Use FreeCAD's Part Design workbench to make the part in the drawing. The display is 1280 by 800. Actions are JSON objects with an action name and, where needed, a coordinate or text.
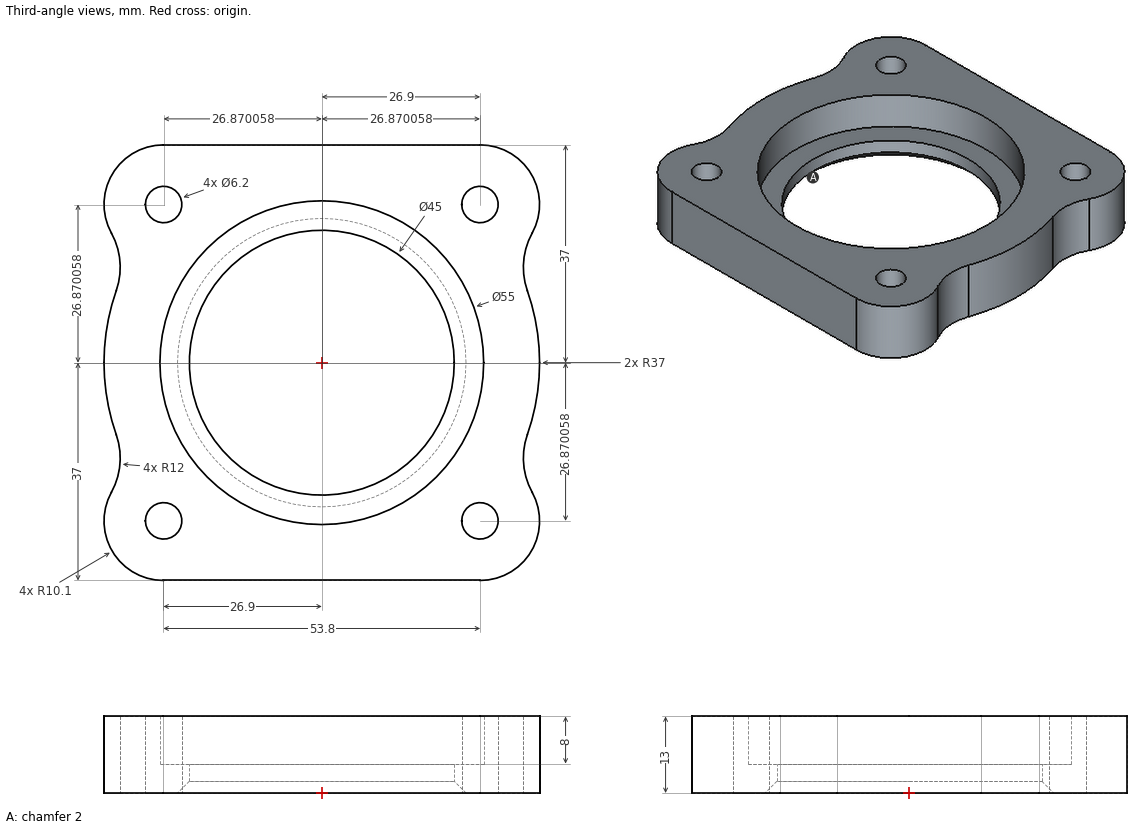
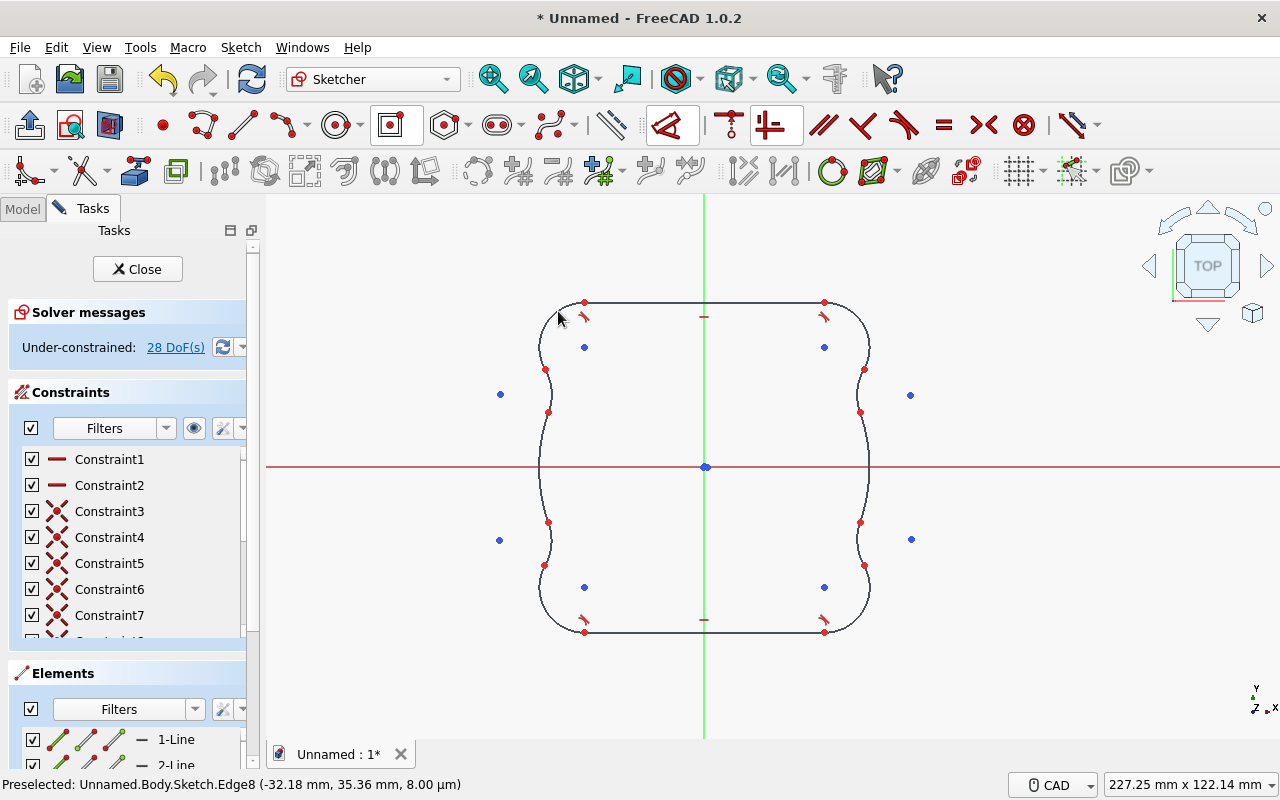
{"action": "left_click", "coordinate": [851, 624]}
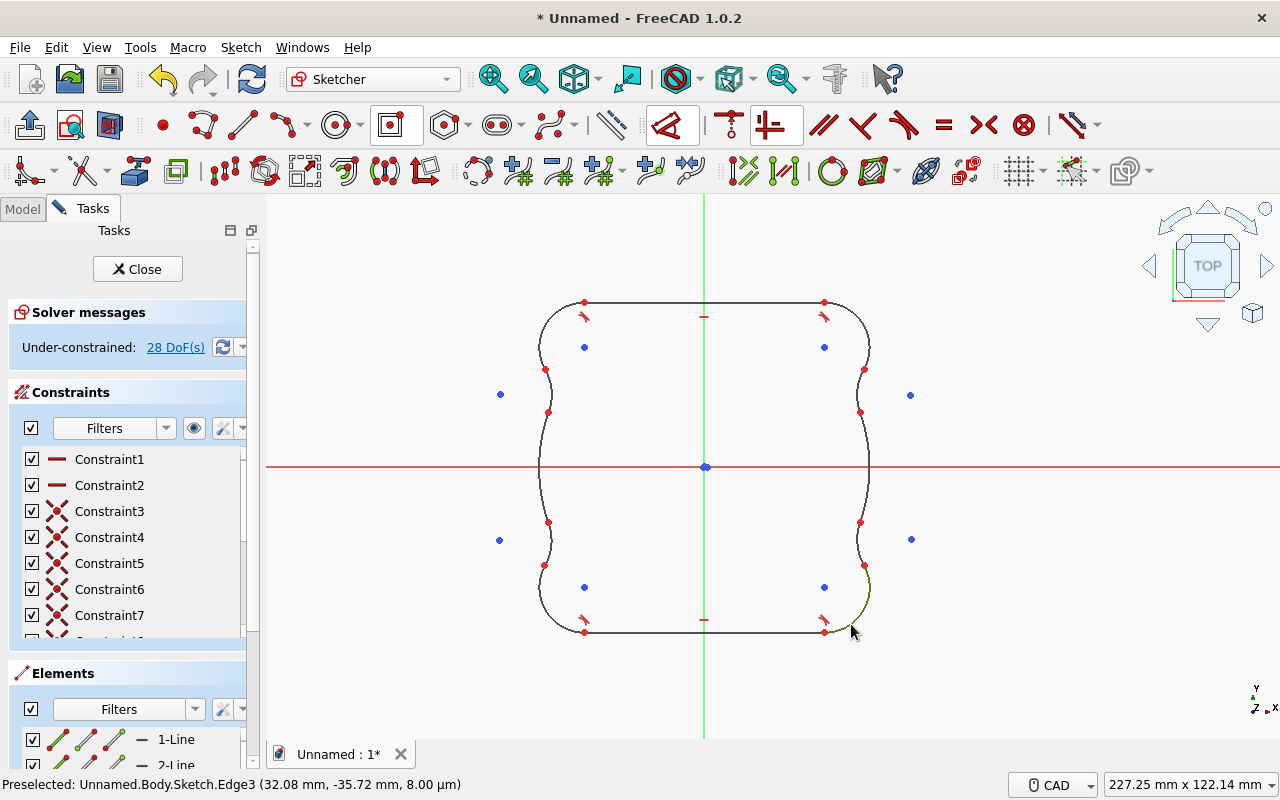
{"action": "left_click", "coordinate": [857, 535]}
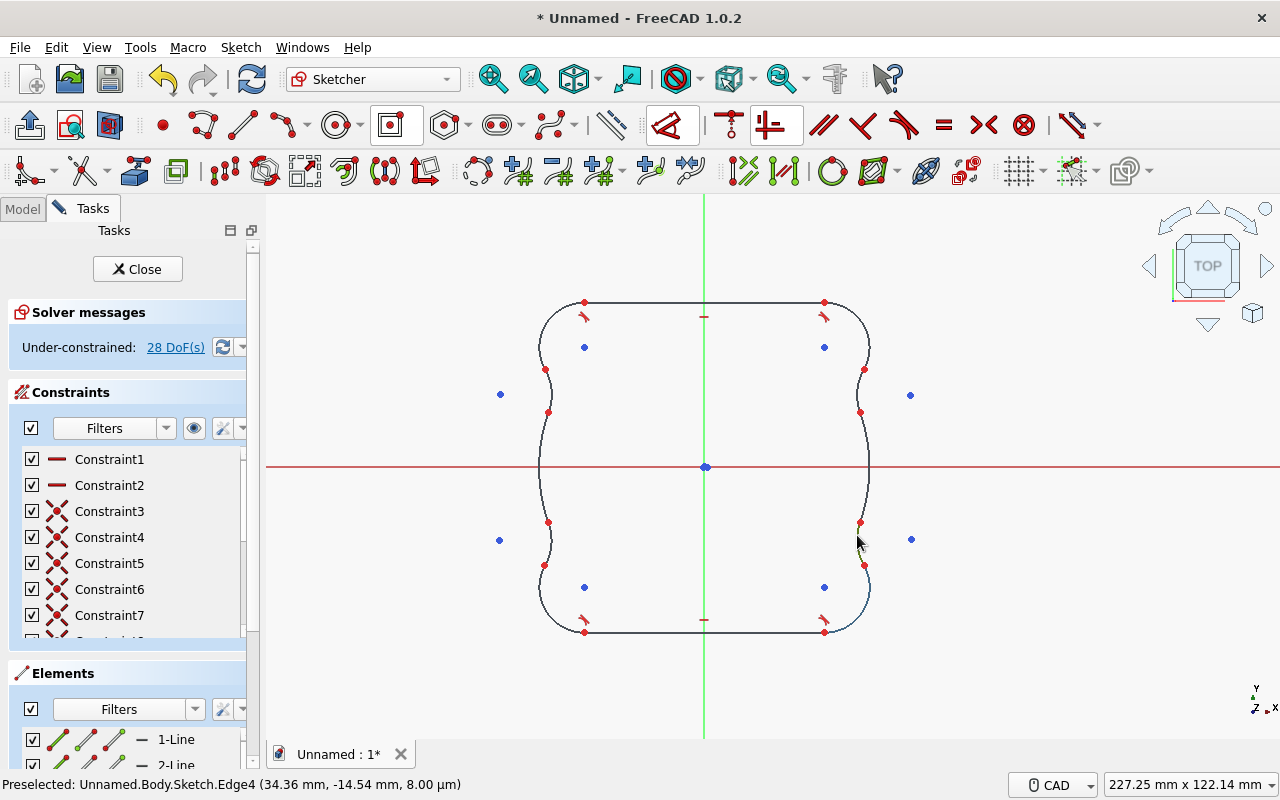
{"action": "key", "text": "t"}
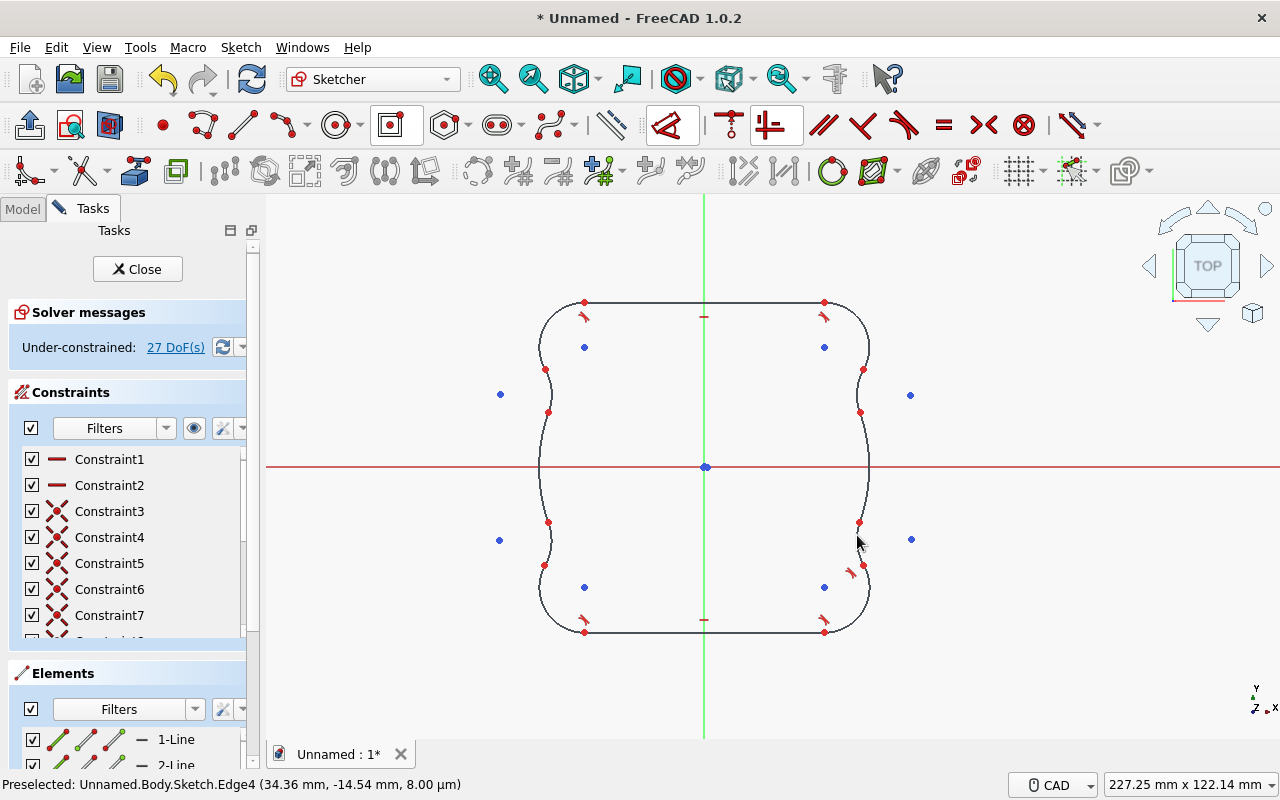
{"action": "left_click", "coordinate": [857, 535]}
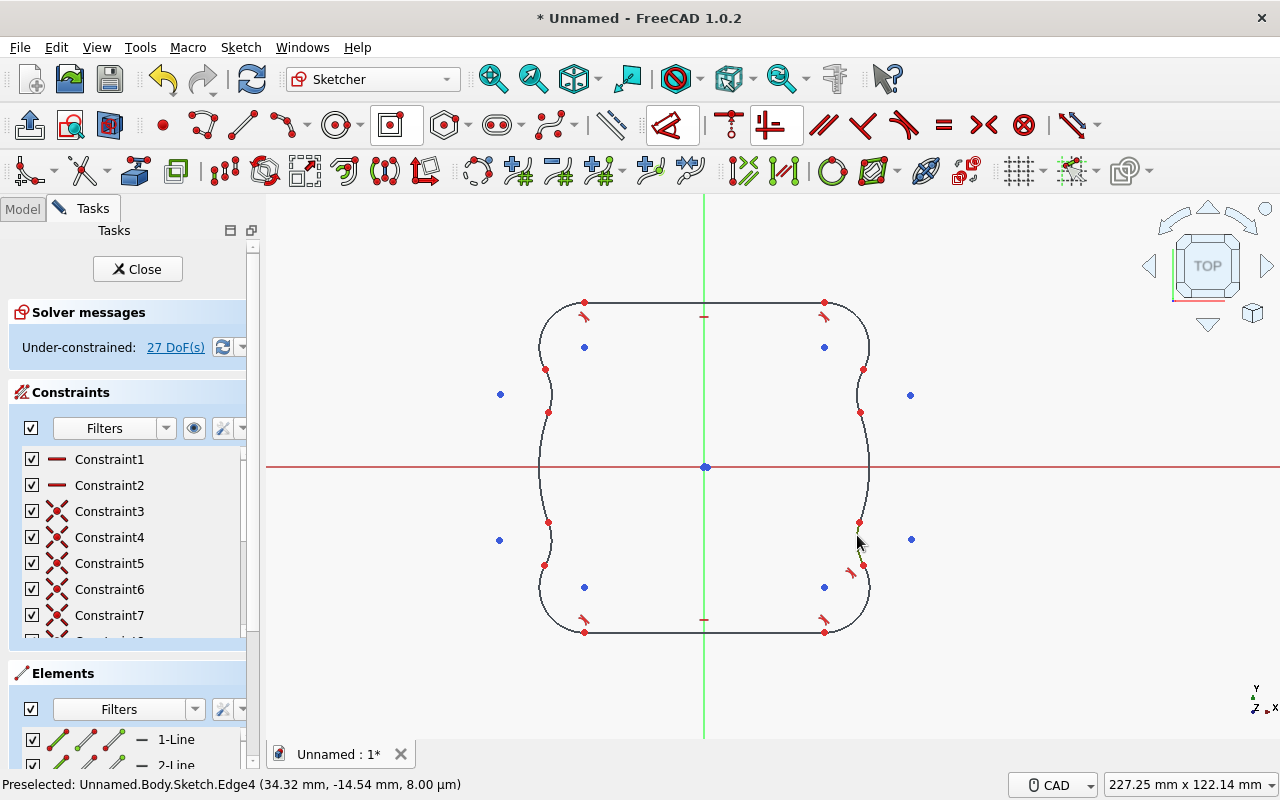
{"action": "left_click", "coordinate": [868, 490]}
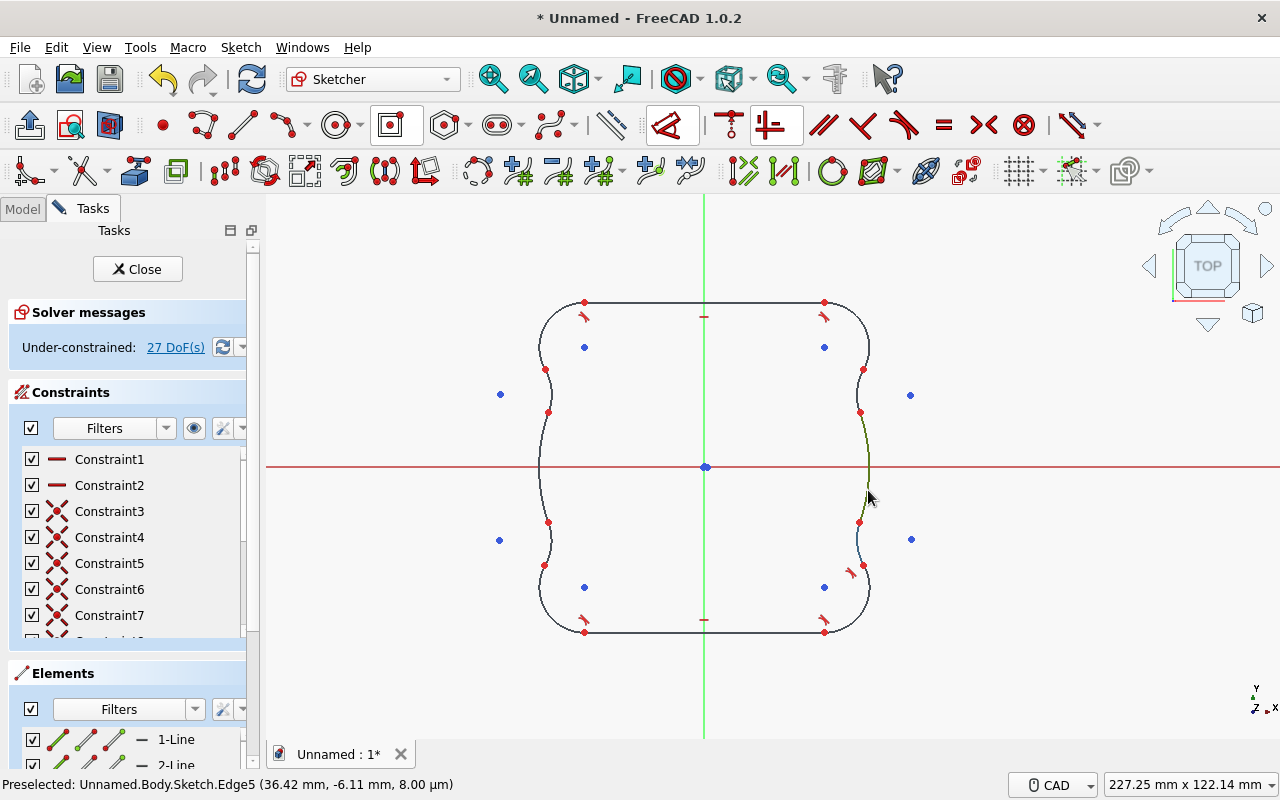
{"action": "key", "text": "t"}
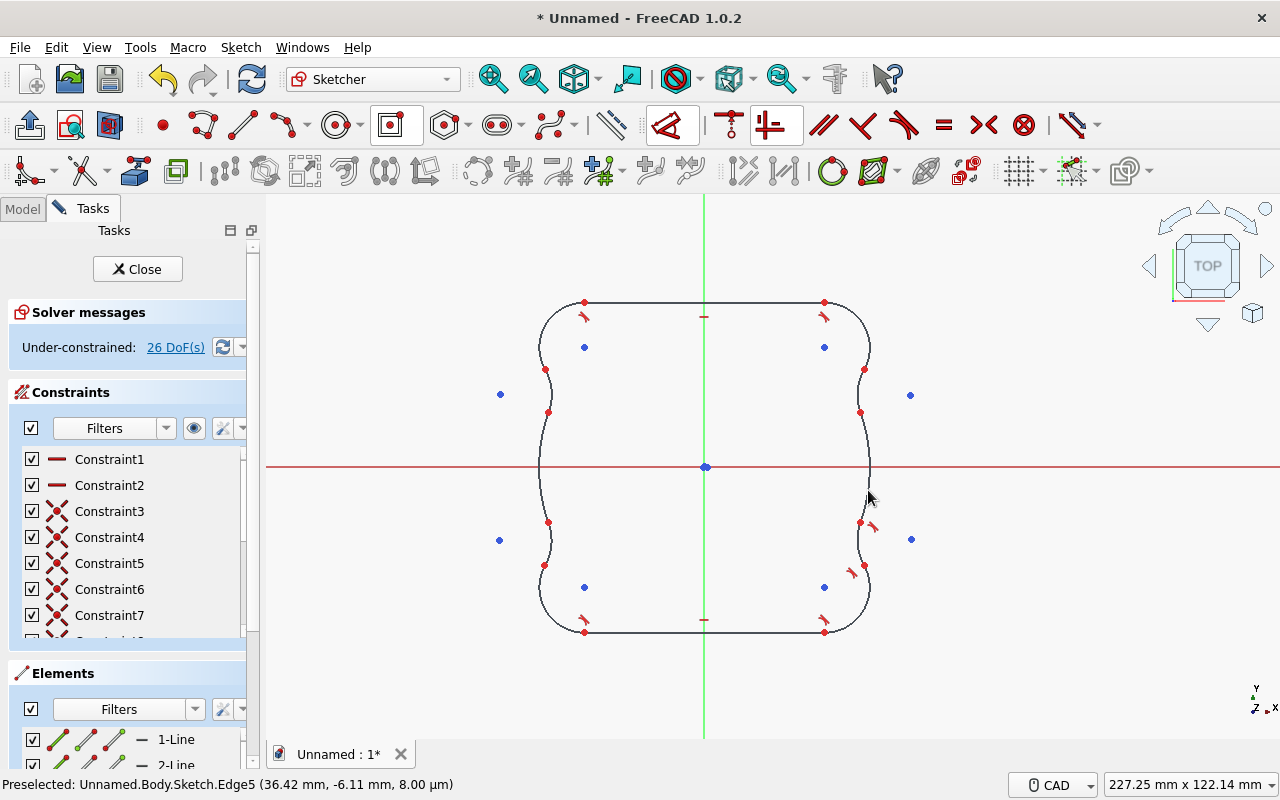
{"action": "left_click", "coordinate": [868, 490]}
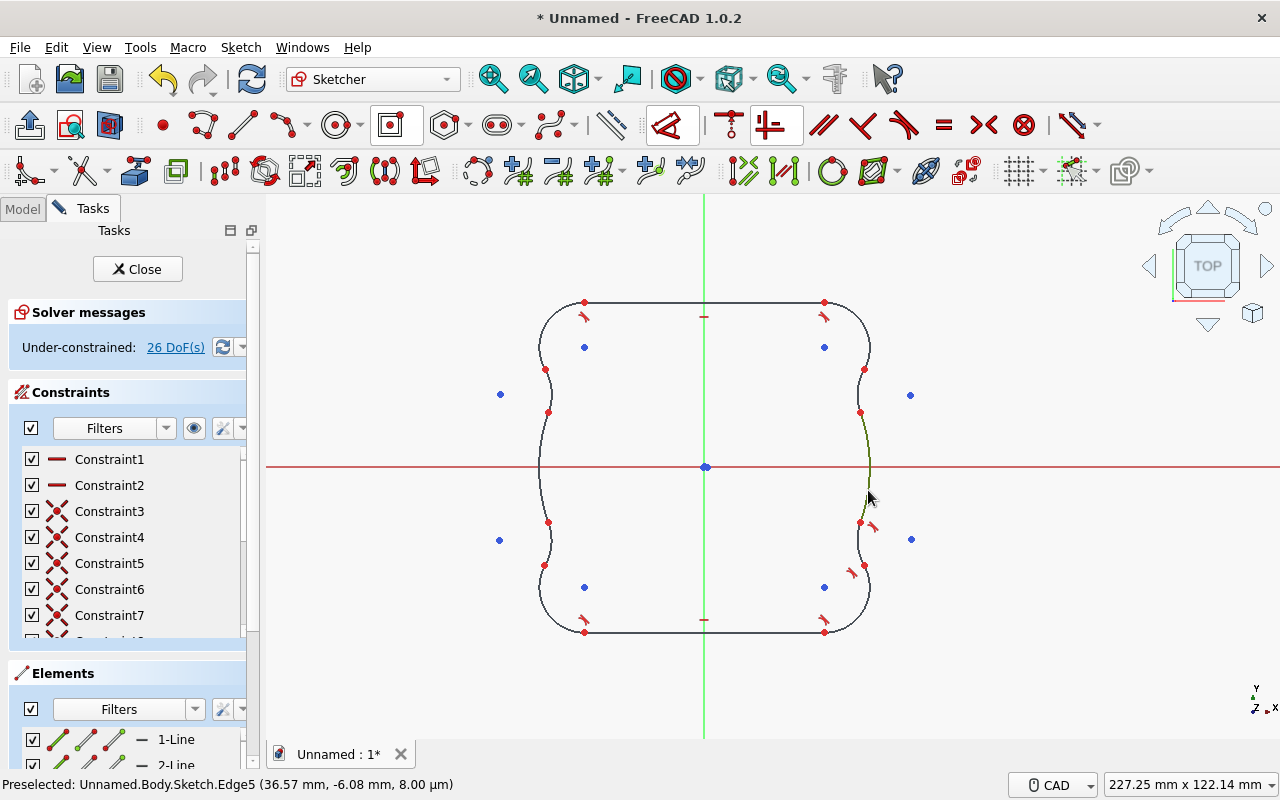
{"action": "left_click", "coordinate": [859, 382]}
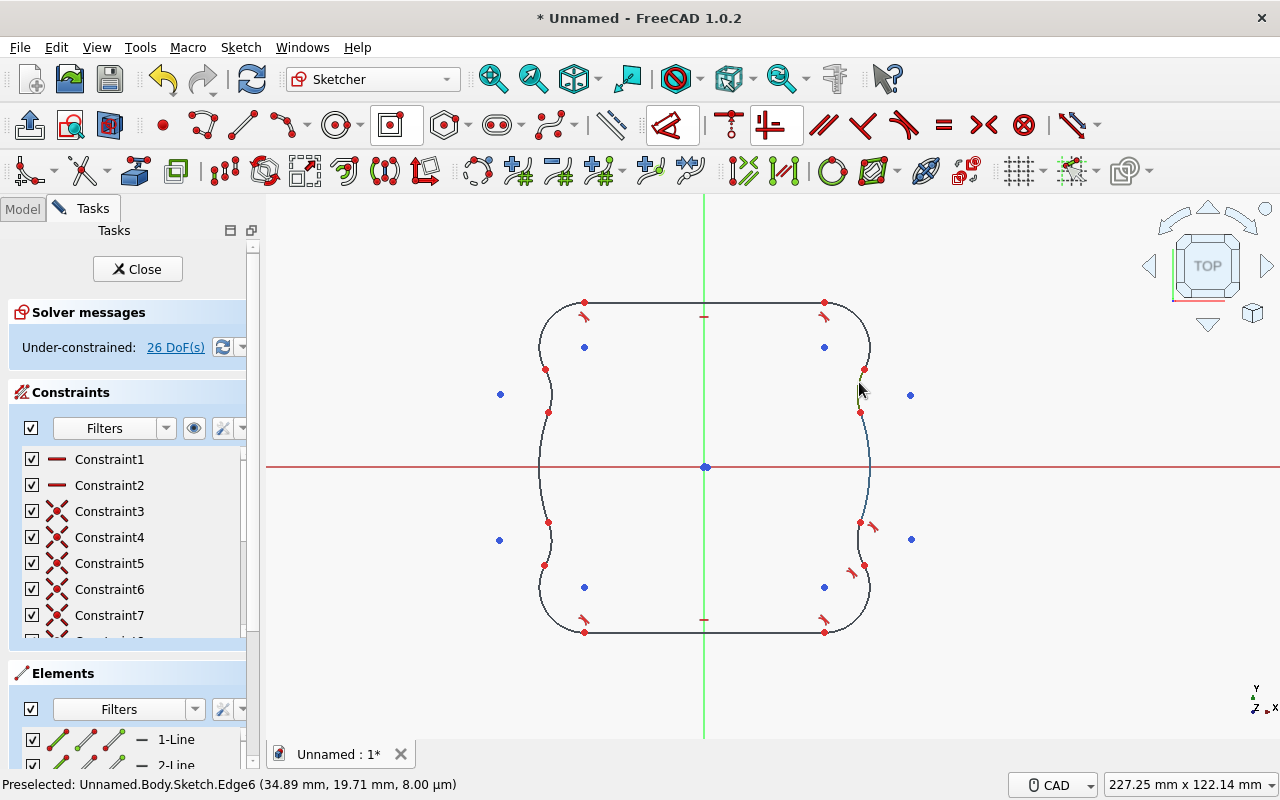
{"action": "left_click", "coordinate": [904, 126]}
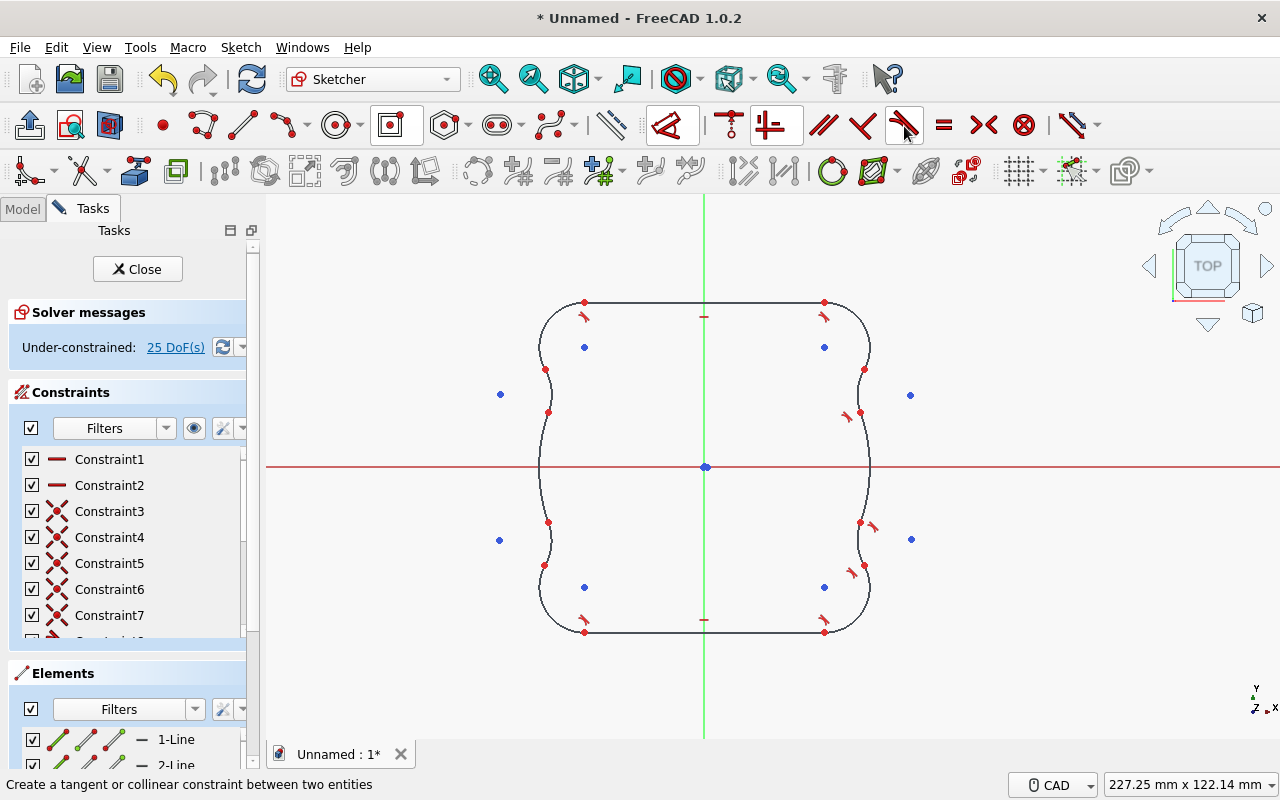
{"action": "left_click", "coordinate": [859, 381]}